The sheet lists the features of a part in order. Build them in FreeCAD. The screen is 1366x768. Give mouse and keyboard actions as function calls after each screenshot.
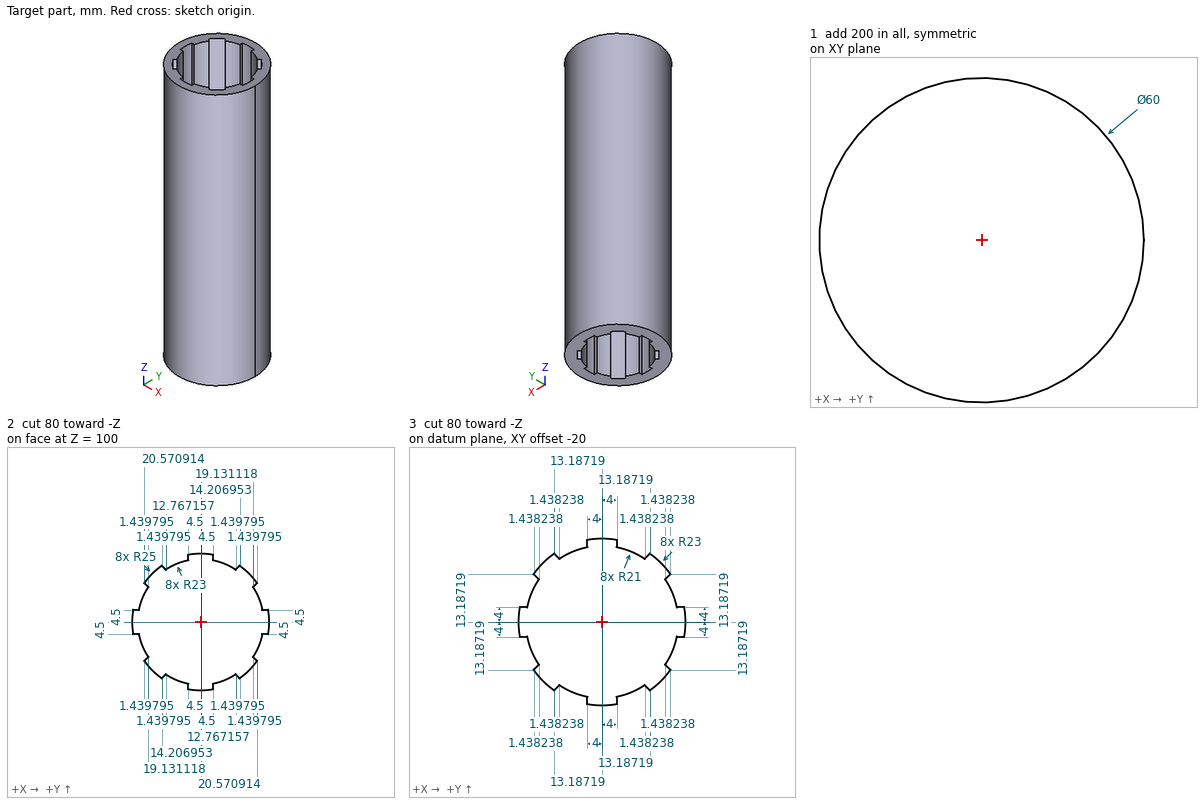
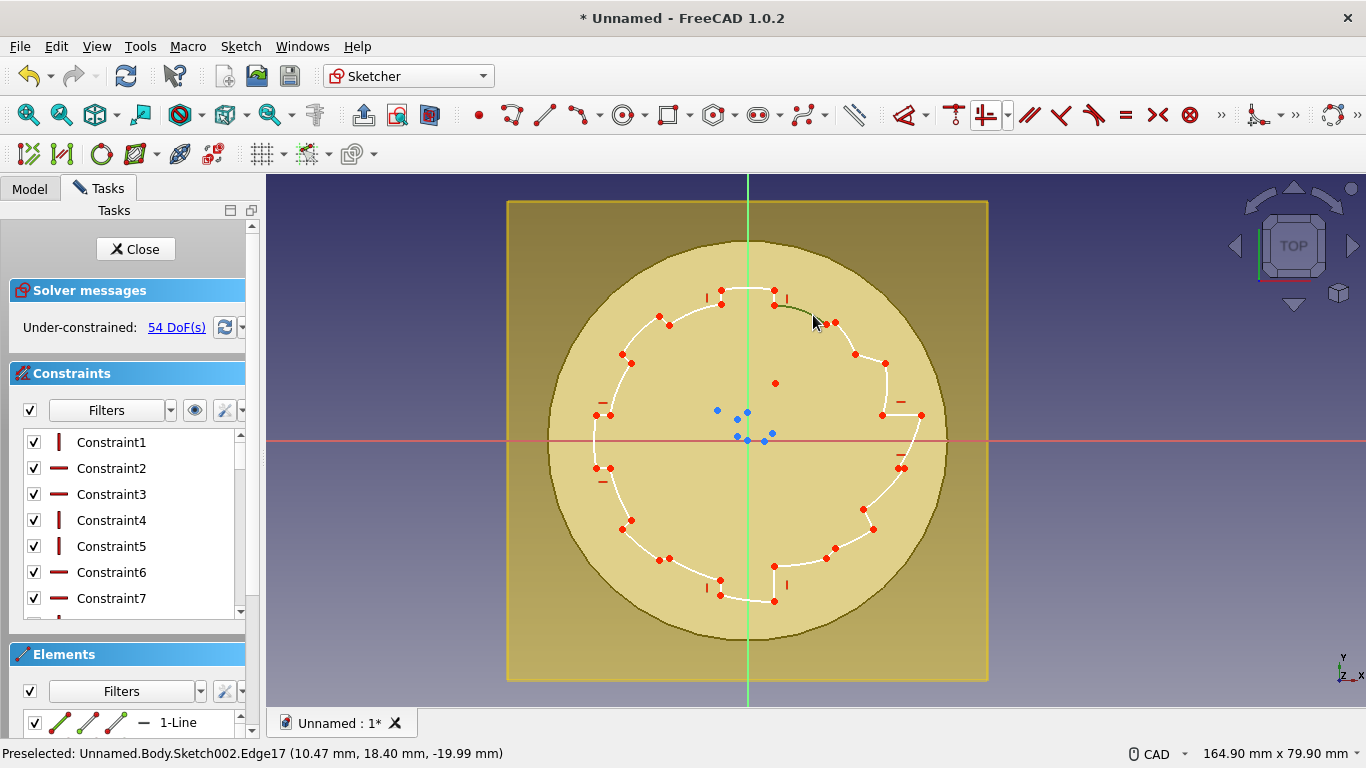
click(615, 485)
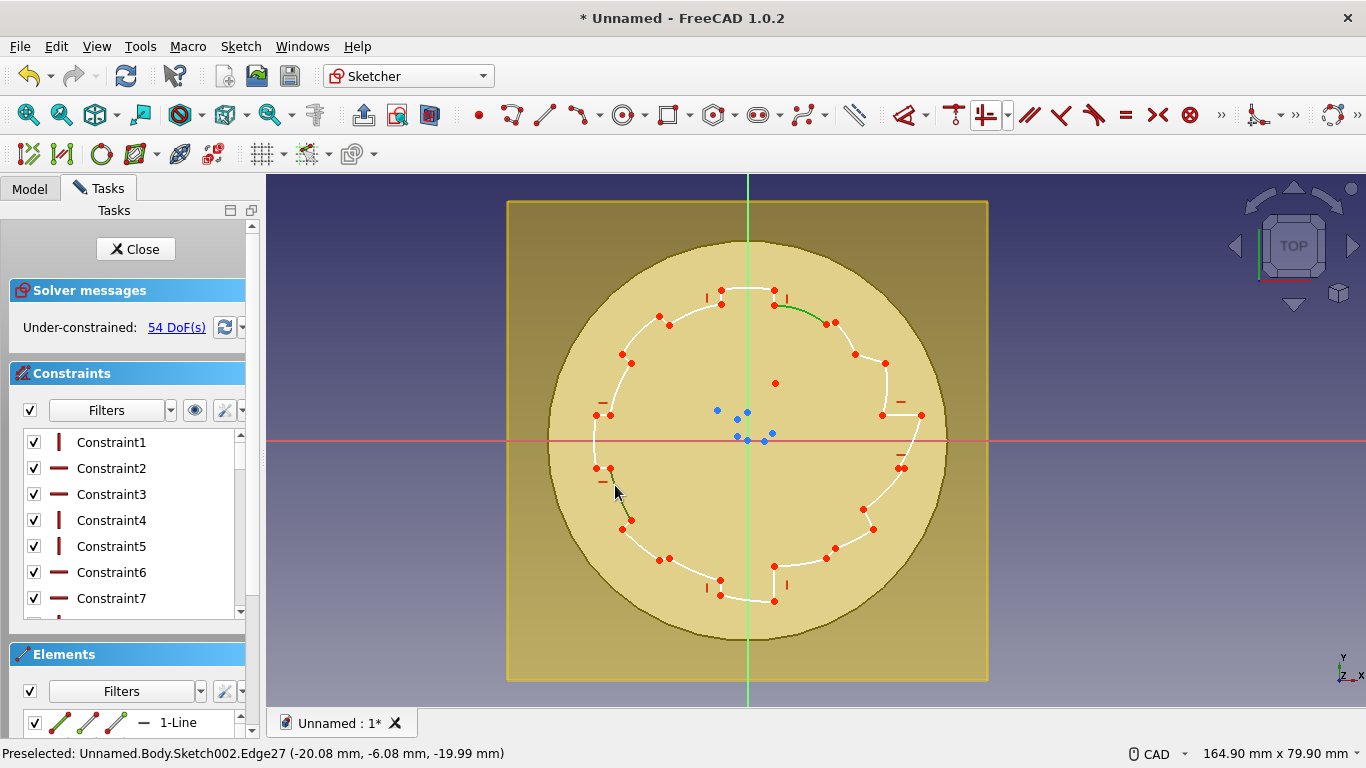
click(954, 116)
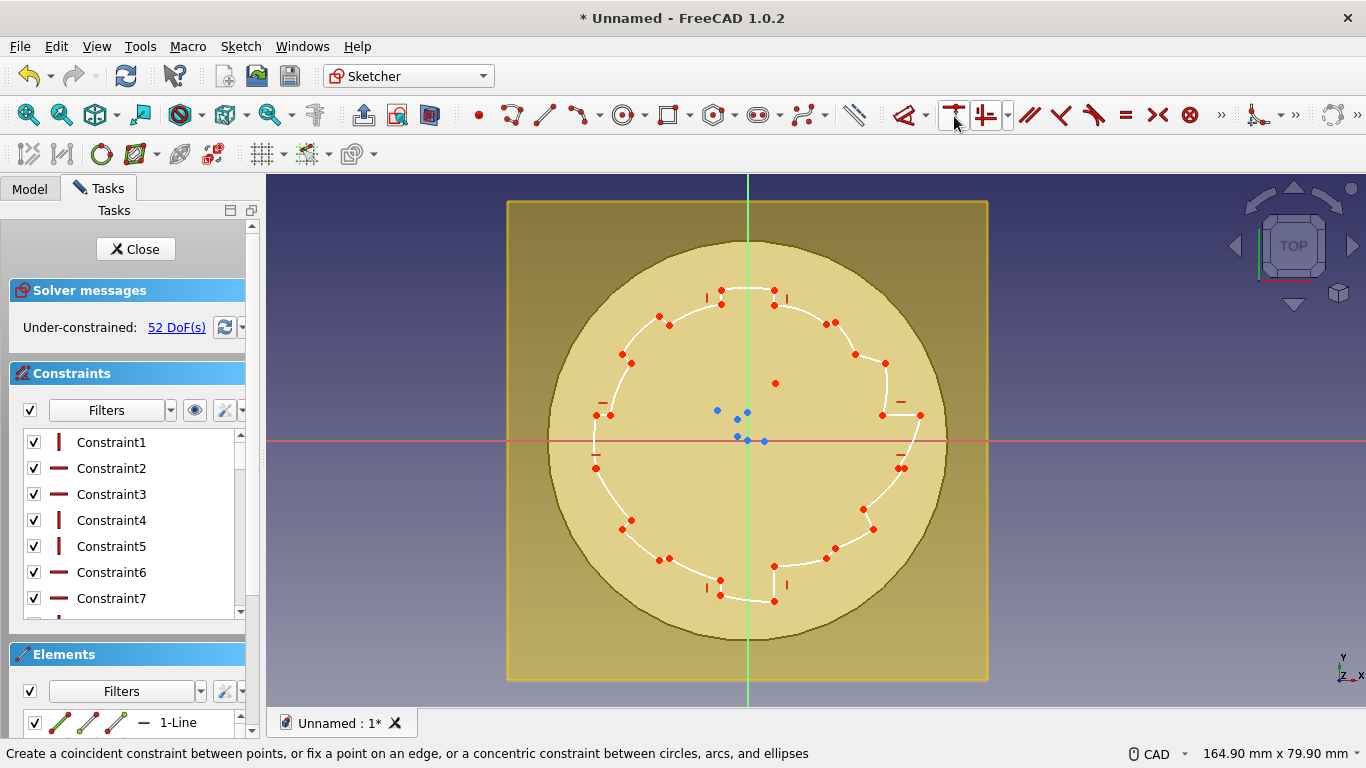
click(813, 315)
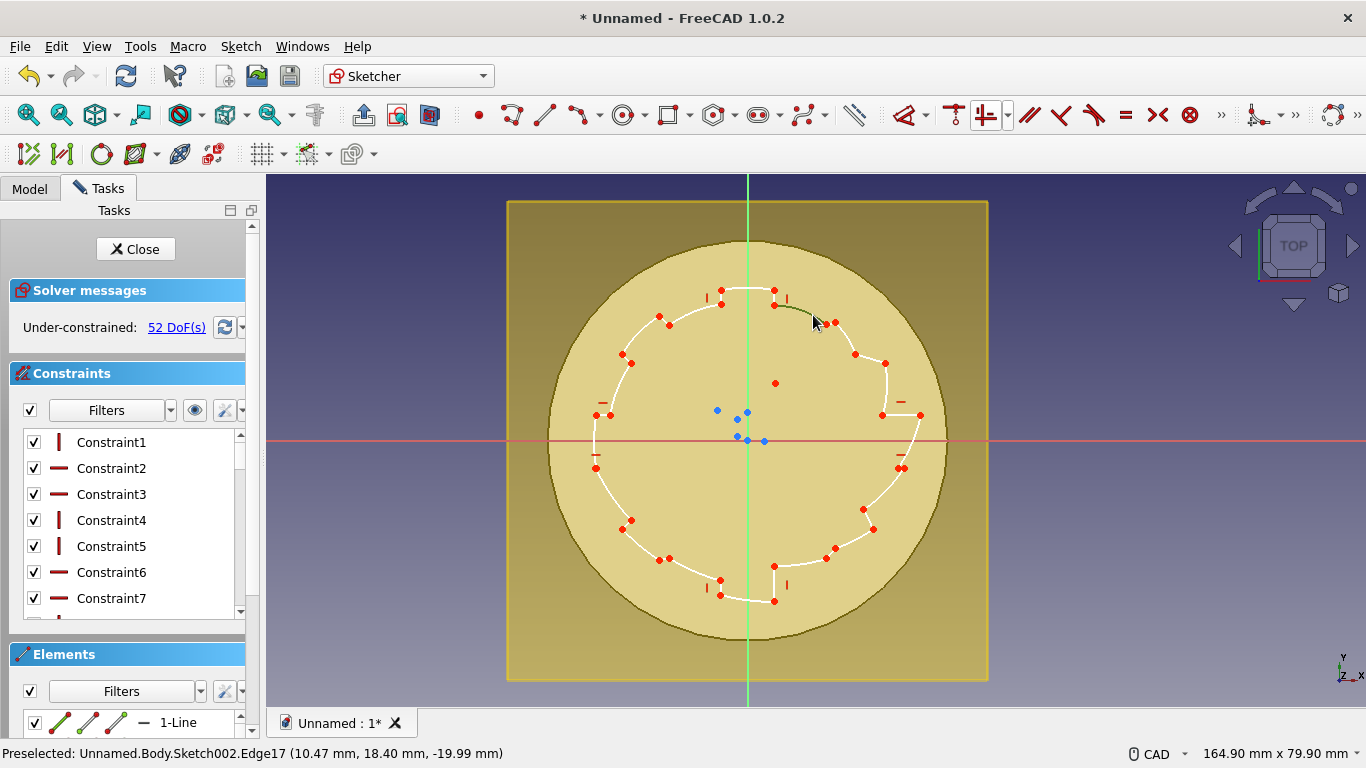
scroll(594, 431, up, 2)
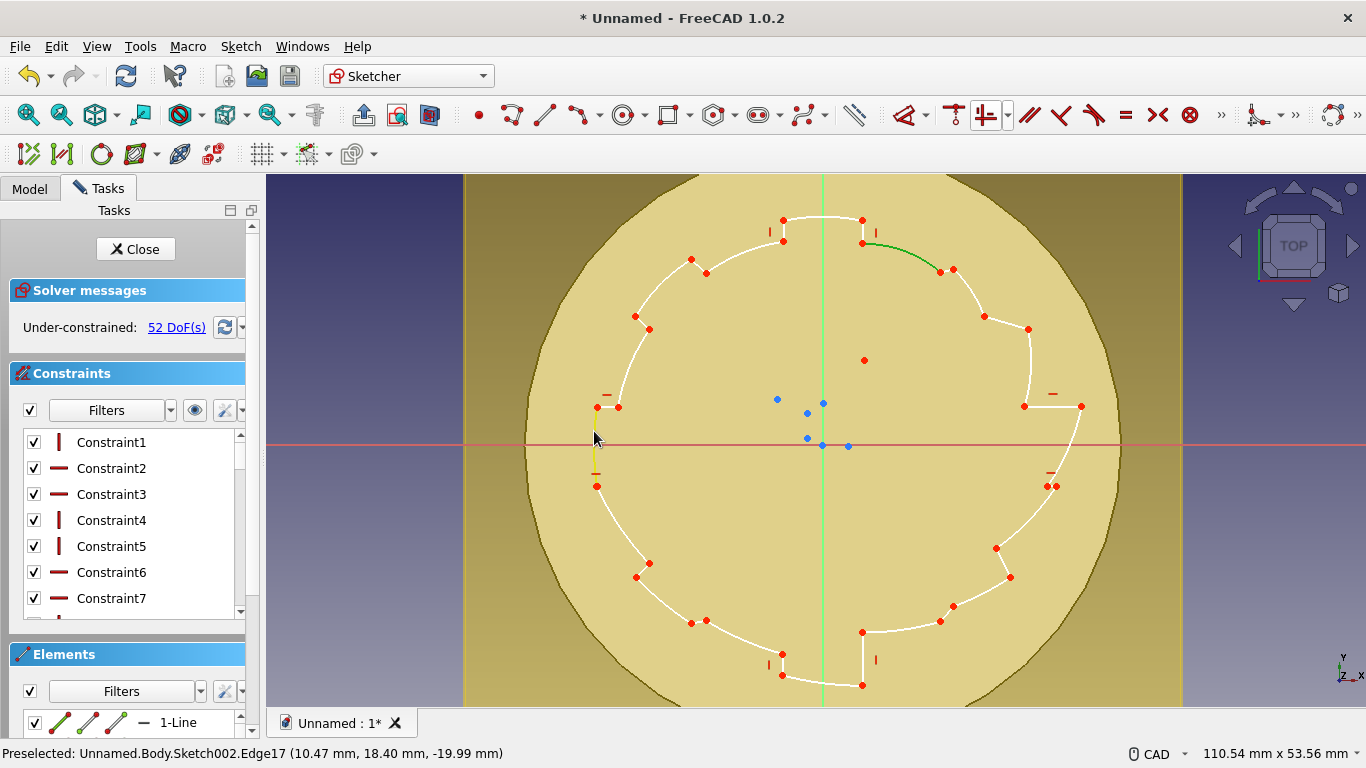
click(595, 431)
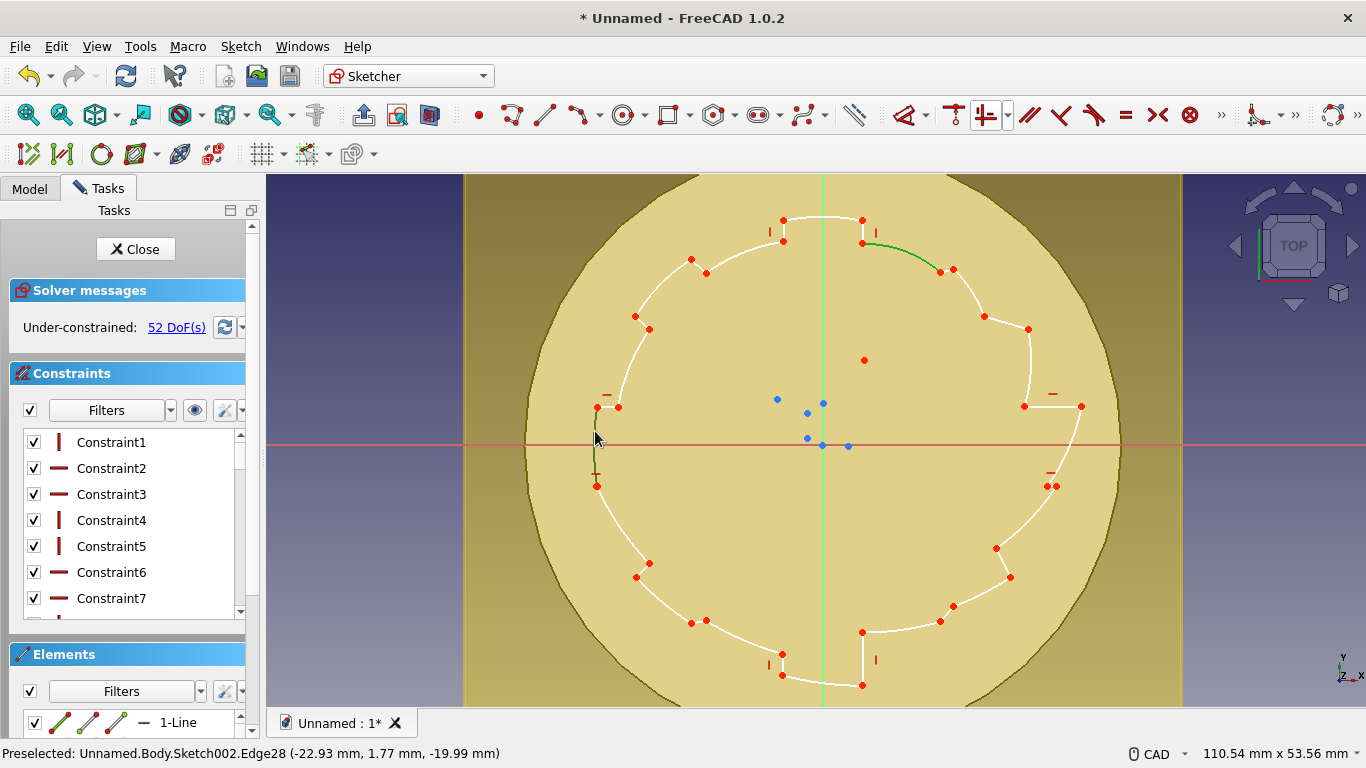
click(954, 116)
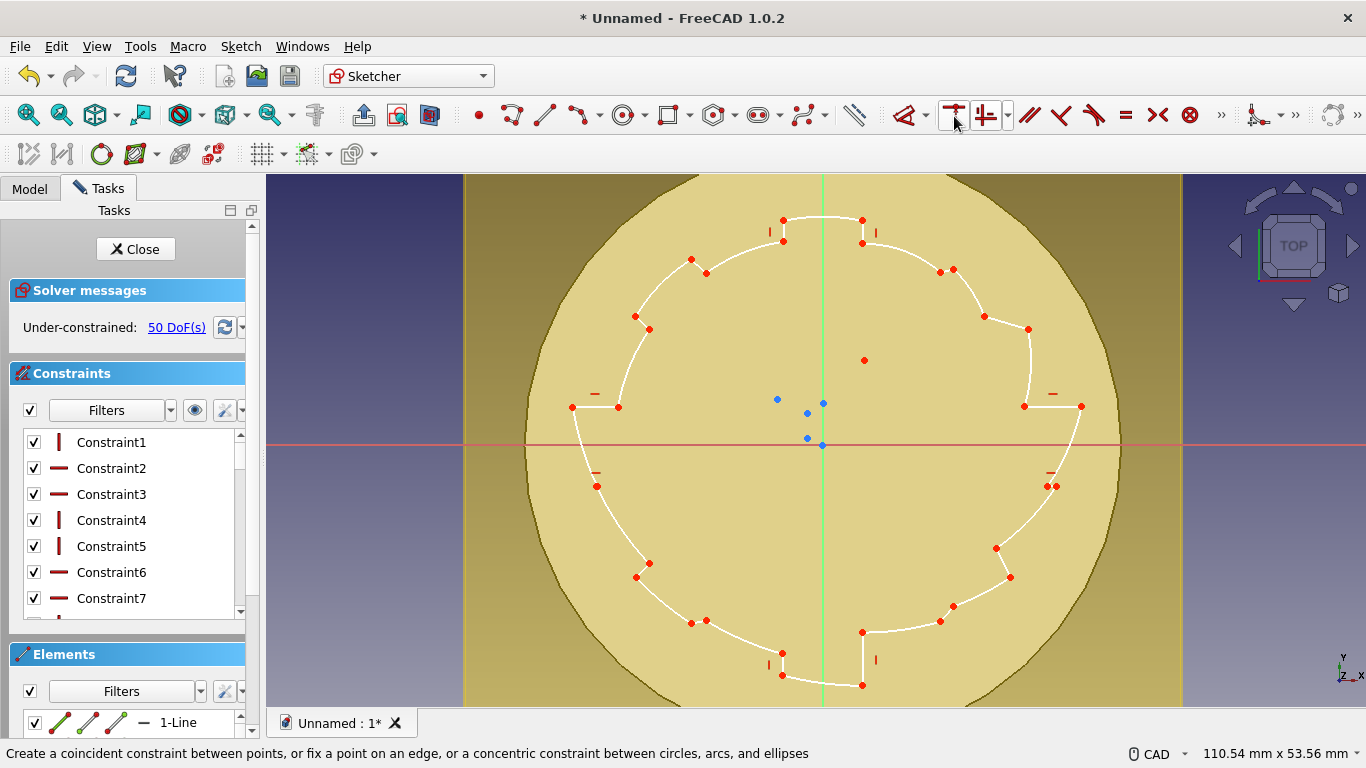
click(920, 258)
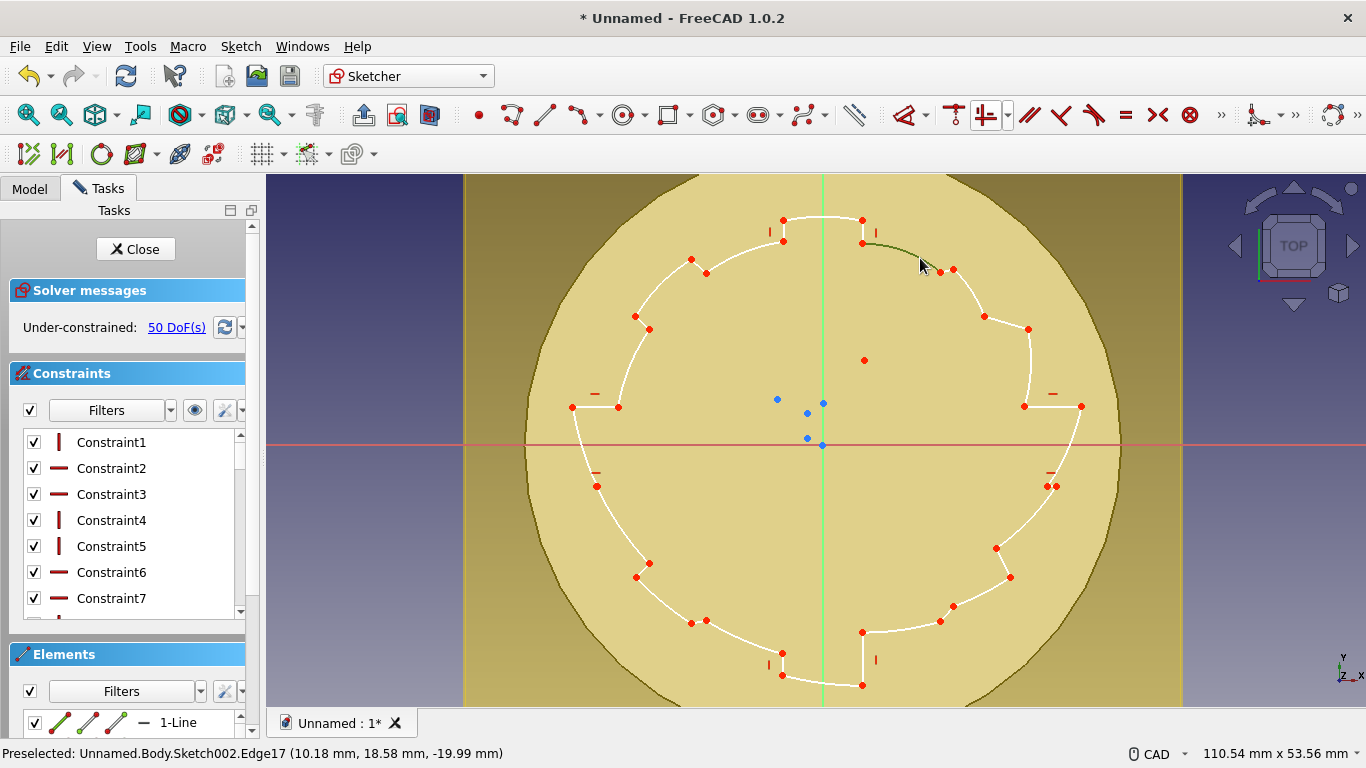
click(636, 352)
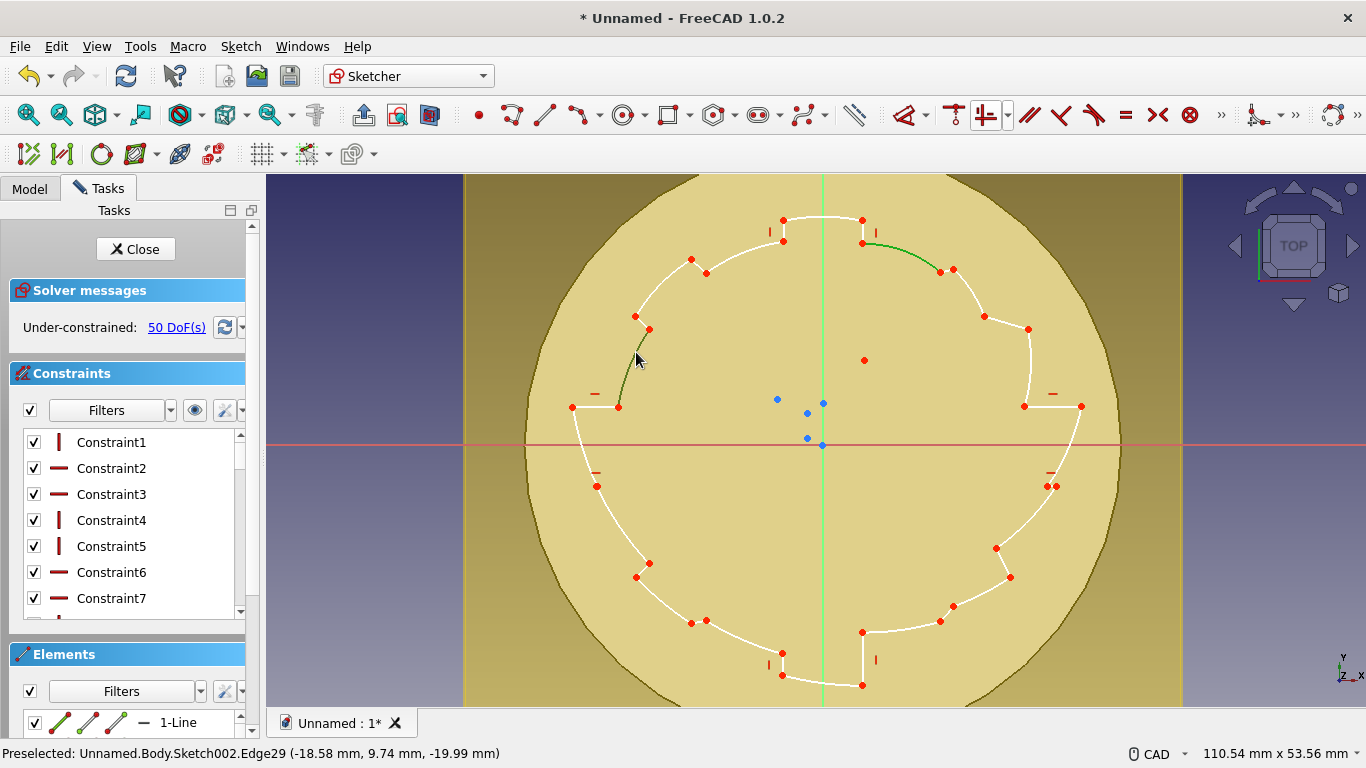
click(954, 116)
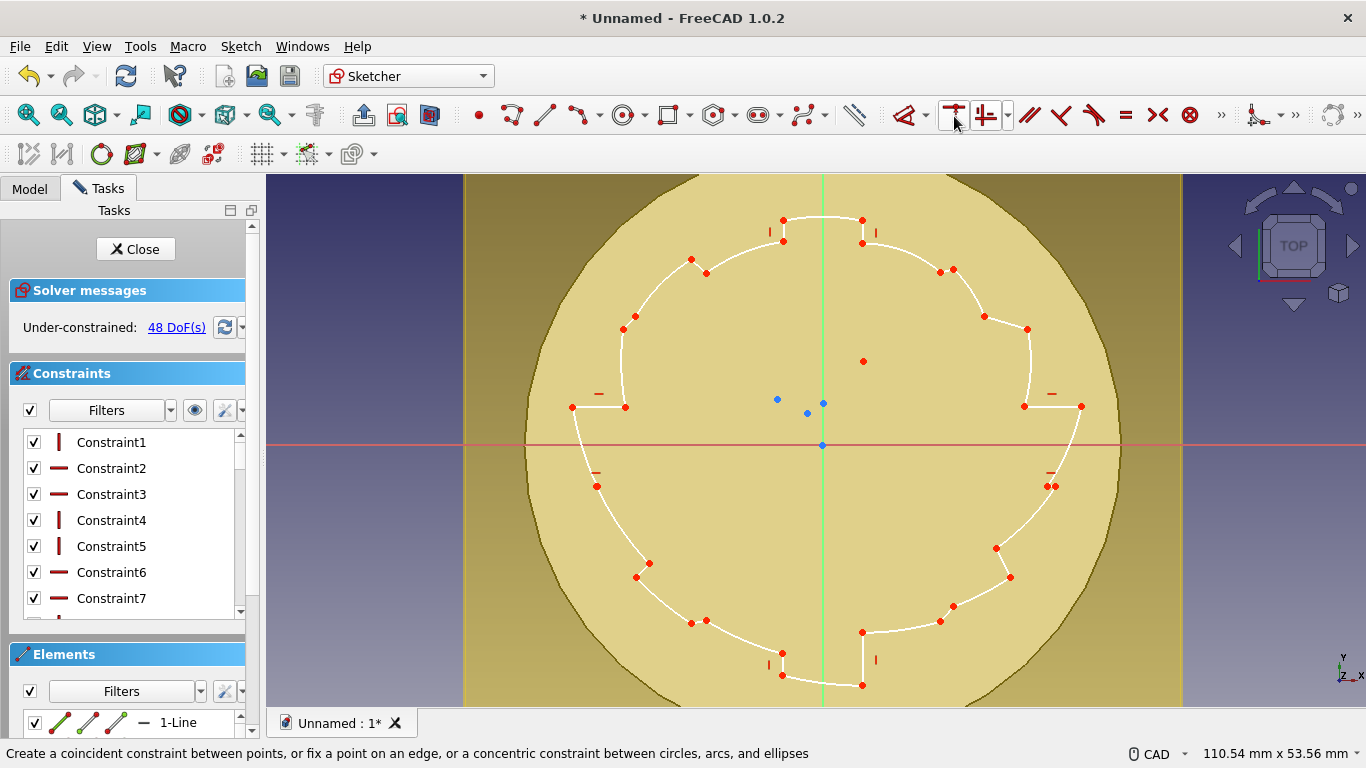
click(920, 258)